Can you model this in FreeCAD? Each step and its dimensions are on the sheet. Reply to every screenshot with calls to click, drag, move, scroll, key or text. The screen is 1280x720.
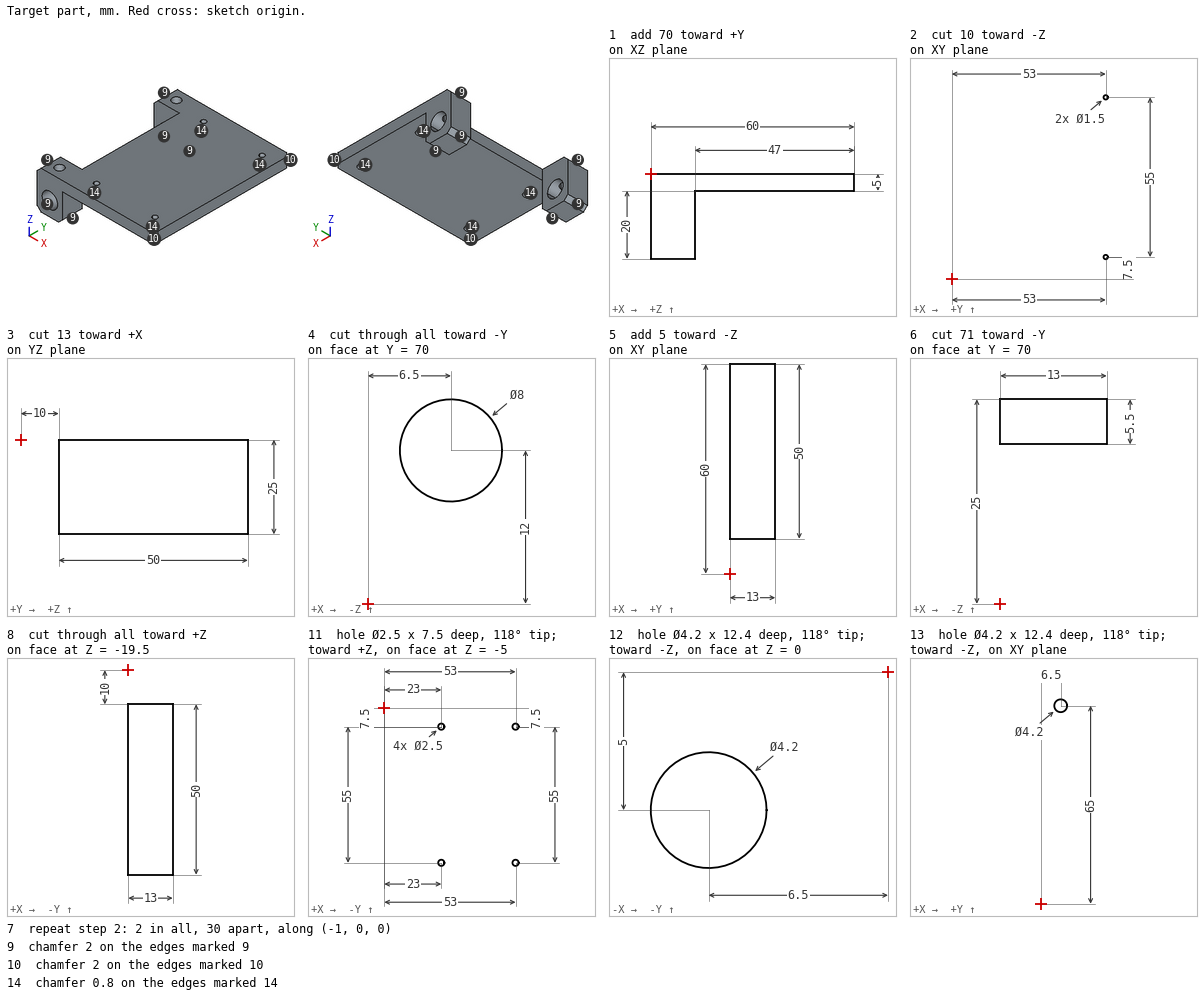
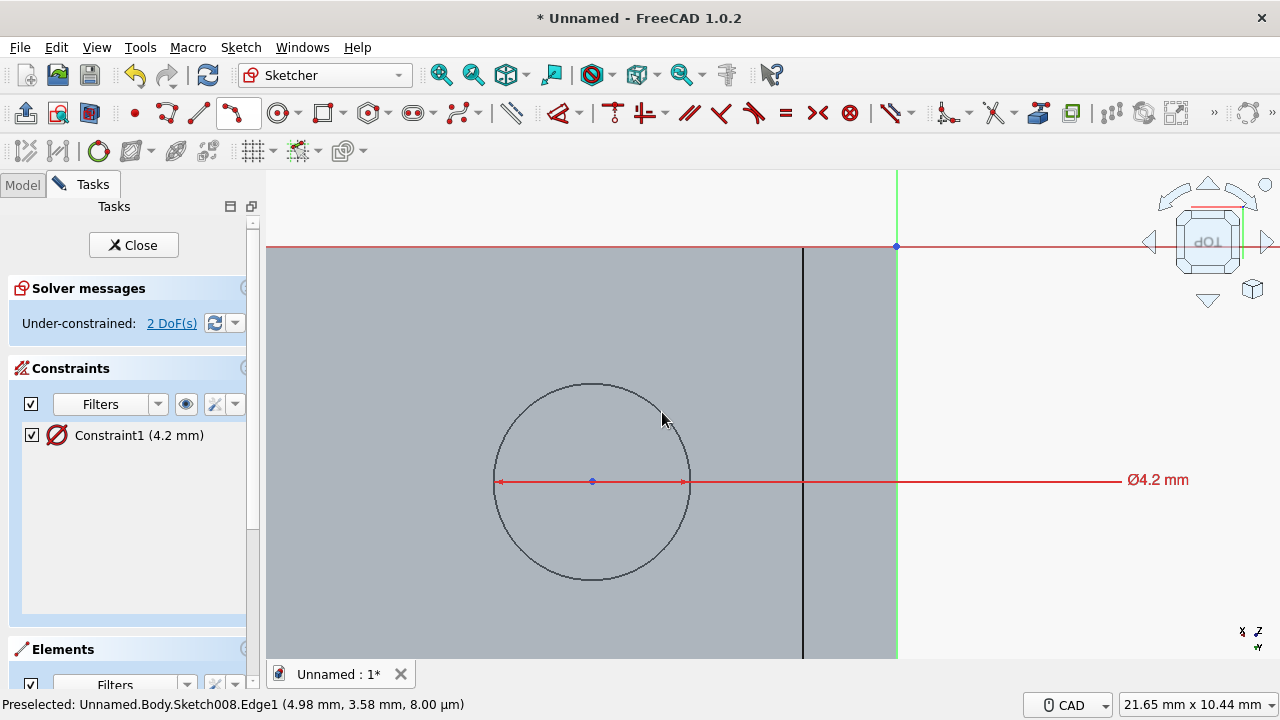
key(d)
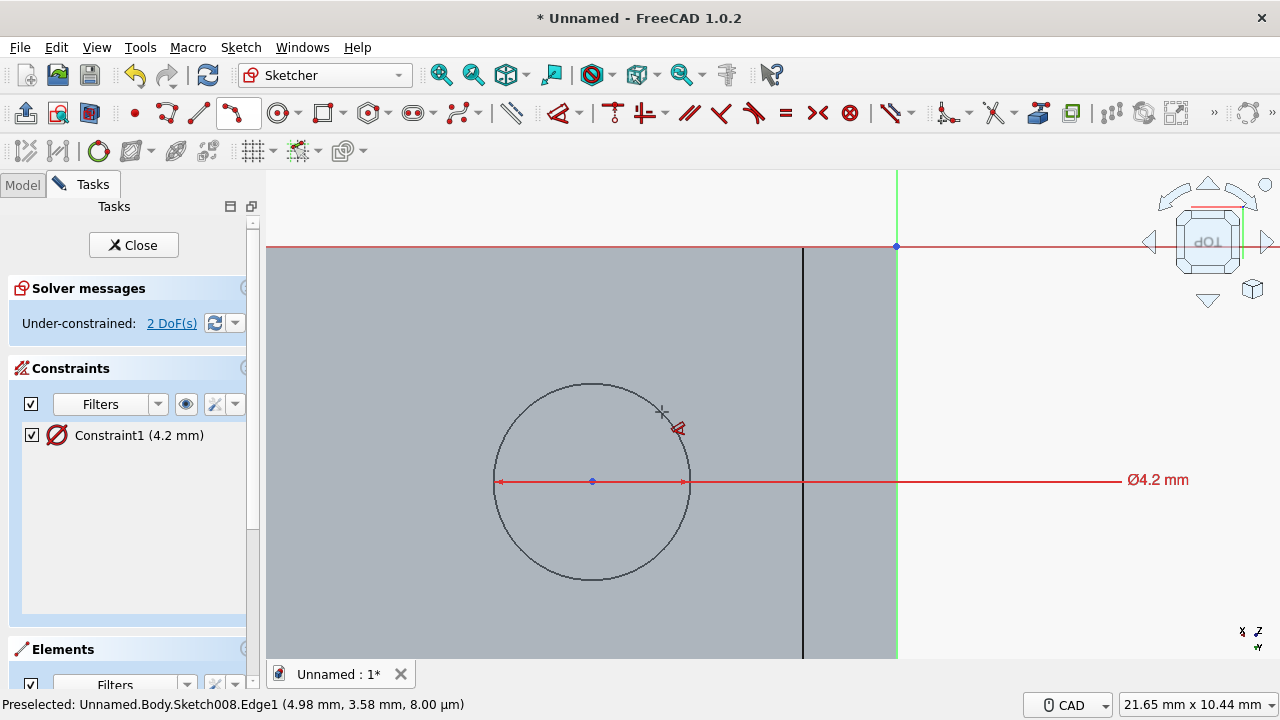
click(592, 482)
click(931, 364)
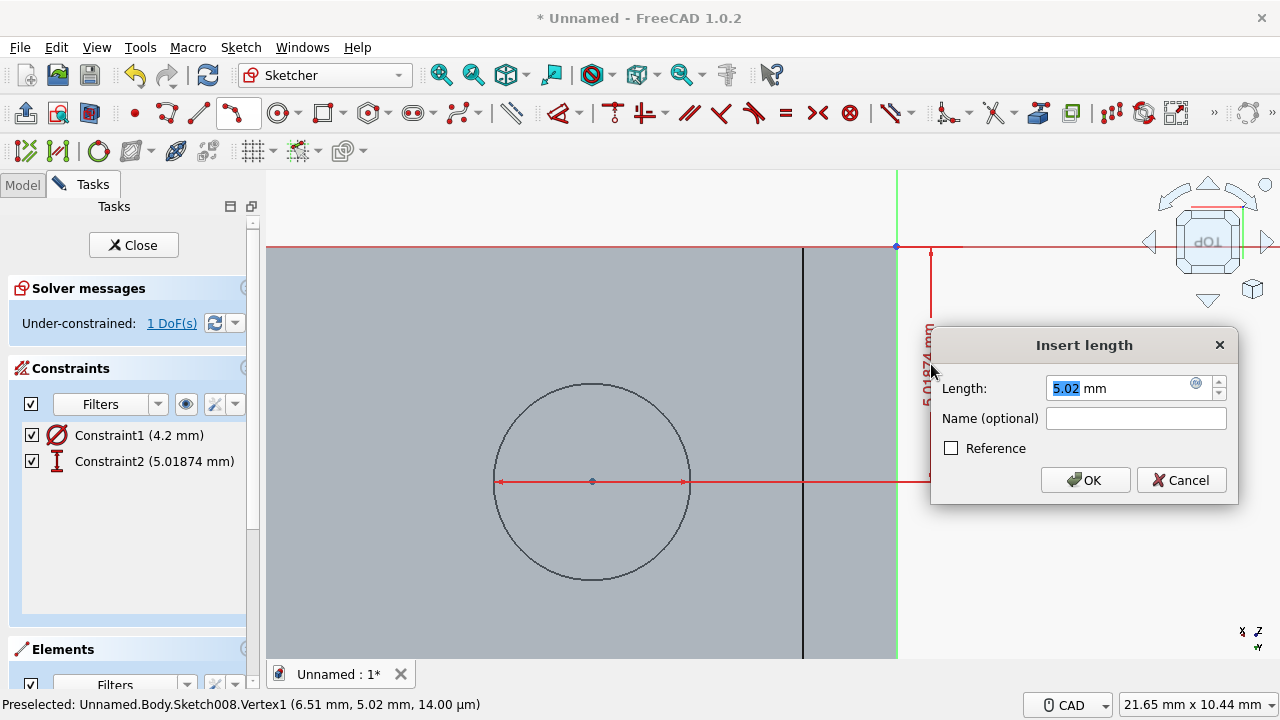
text(5)
key(Return)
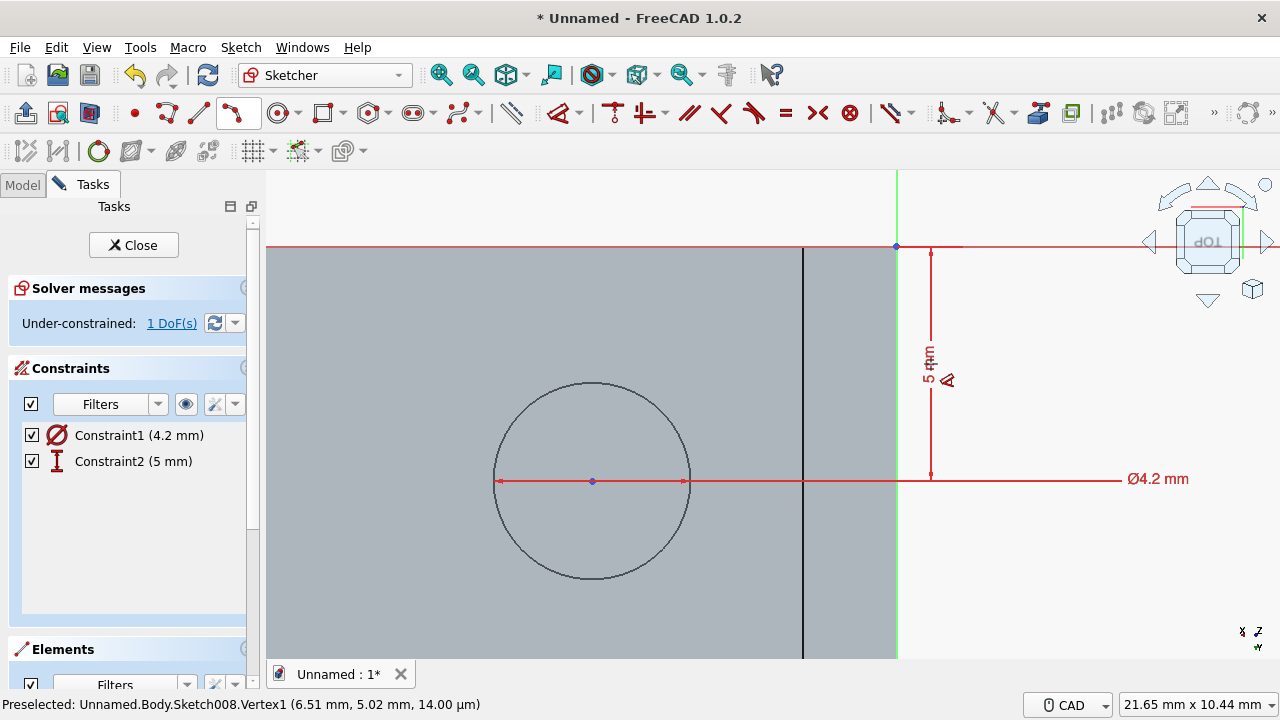
click(592, 481)
click(744, 213)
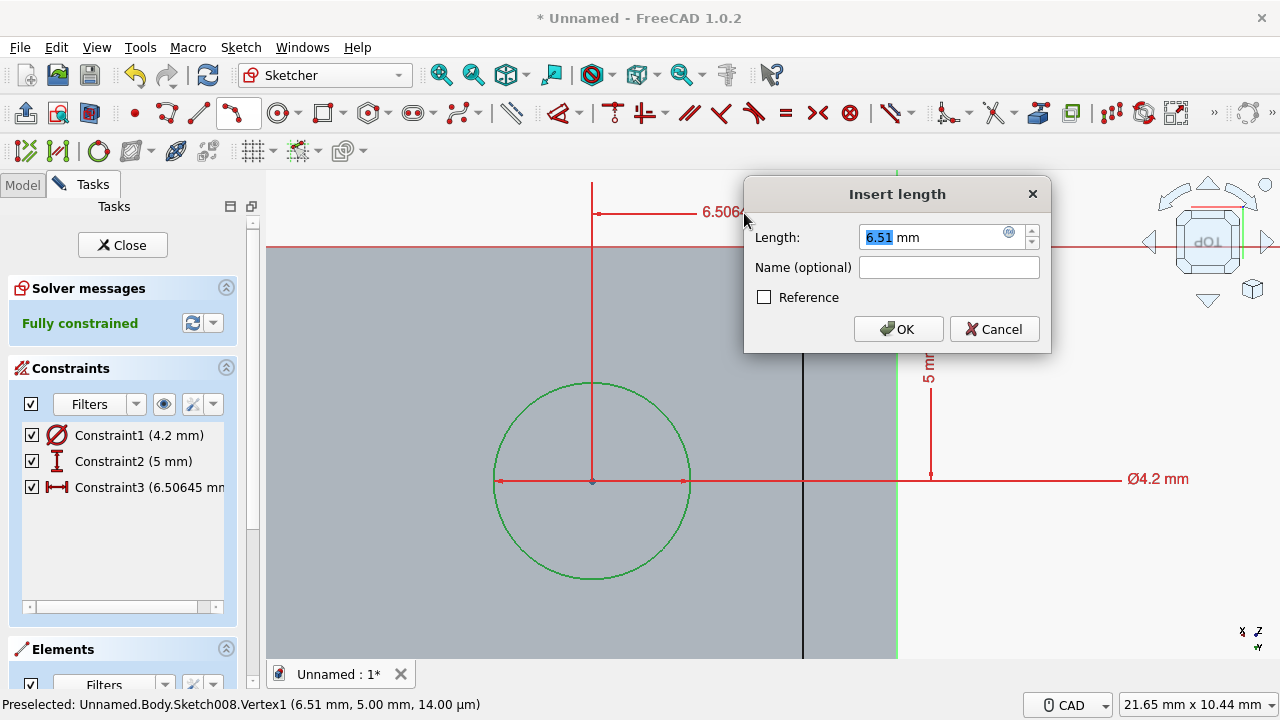
text(6.5)
key(Return)
key(Escape)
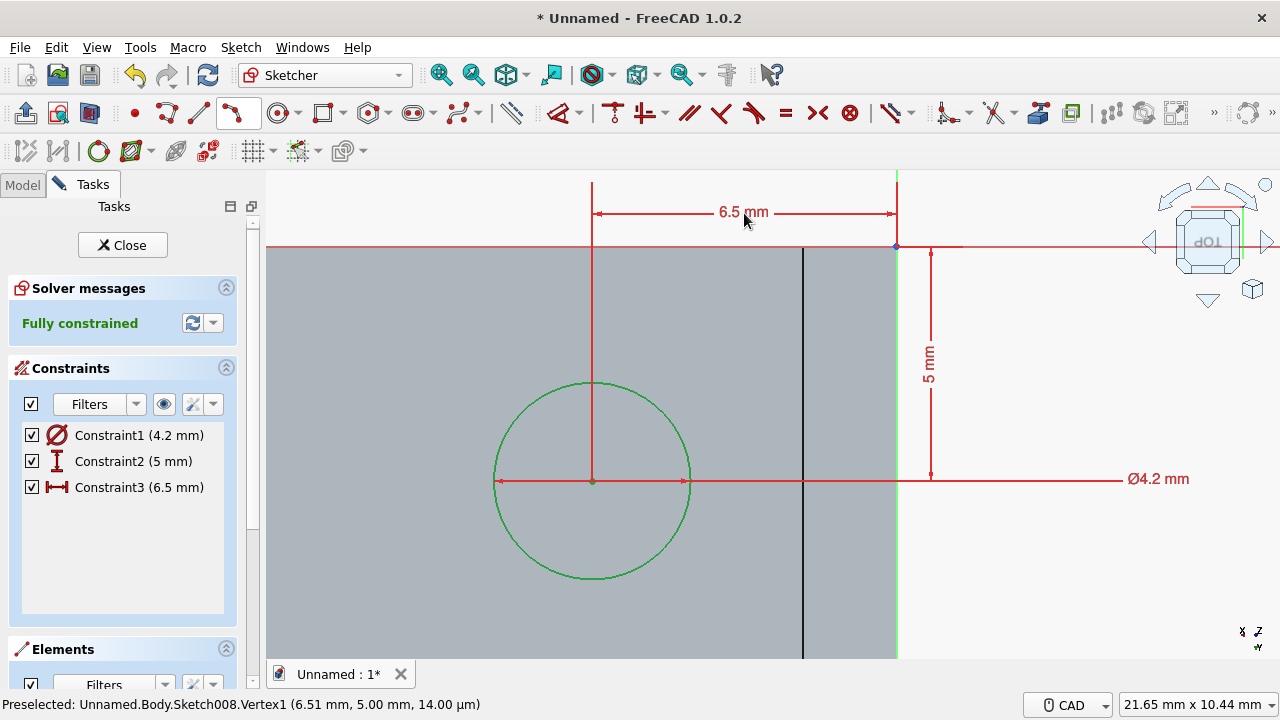
click(123, 245)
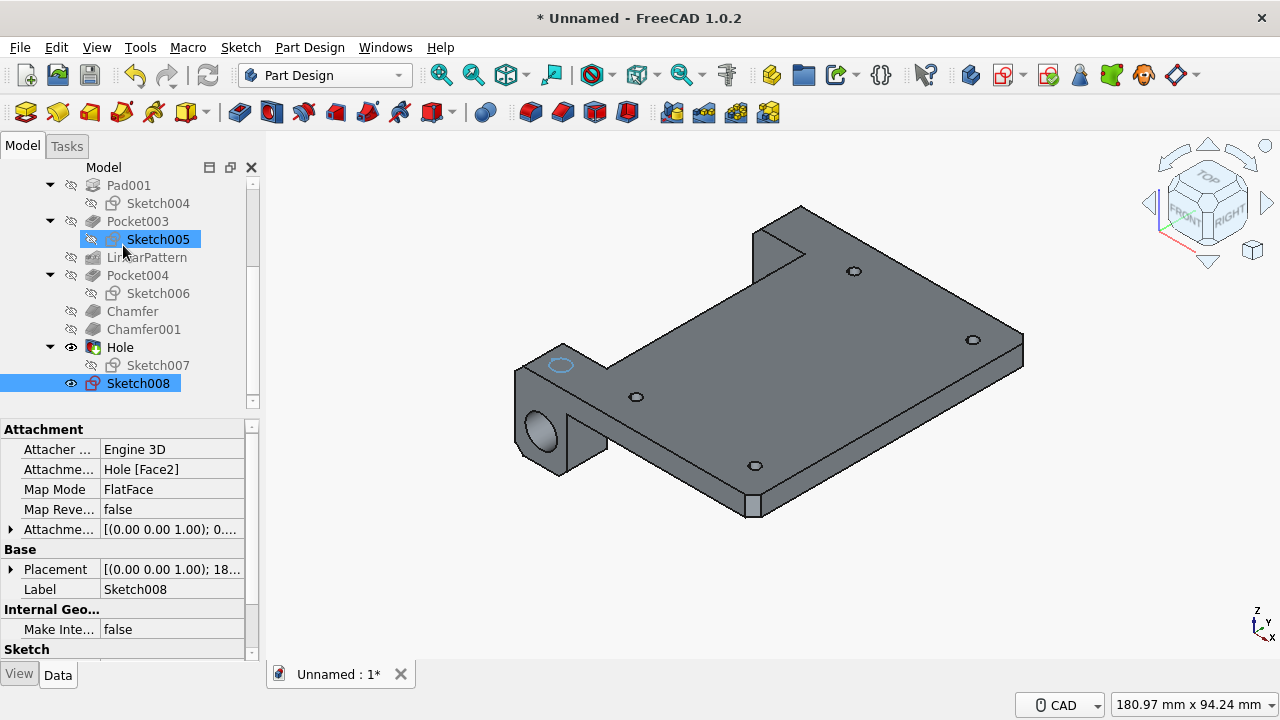
click(272, 112)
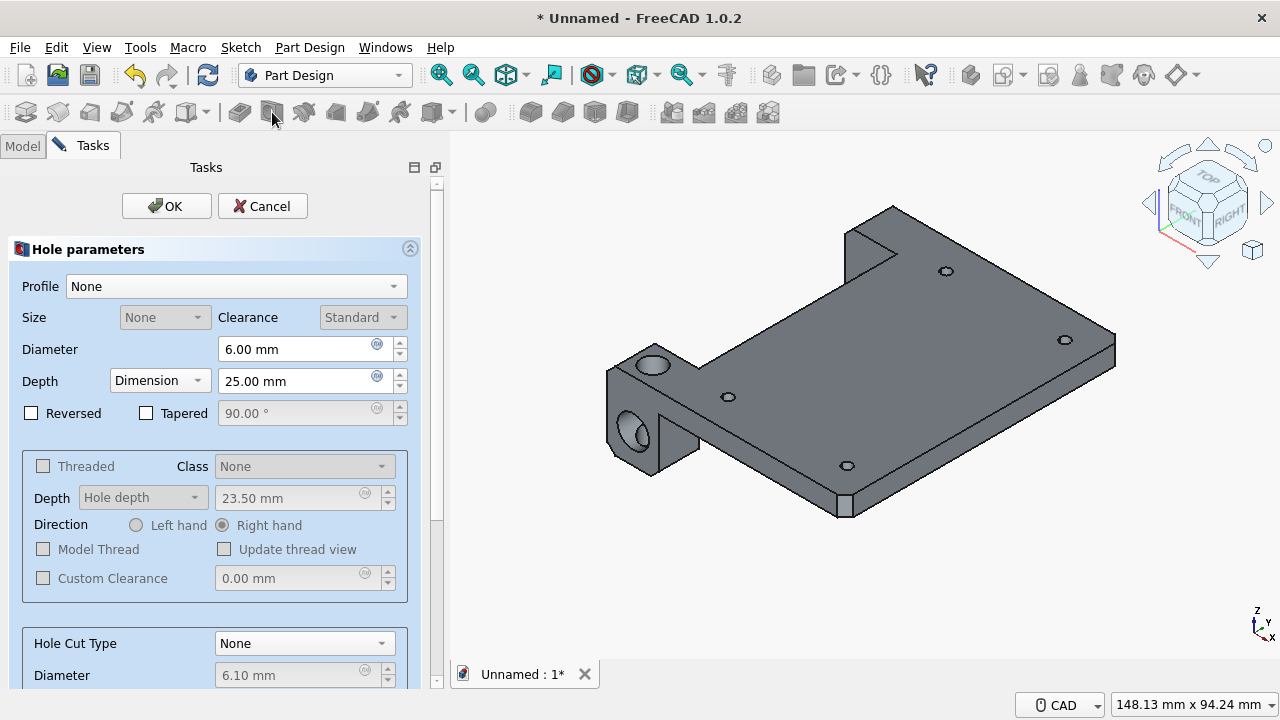
triple_click(305, 349)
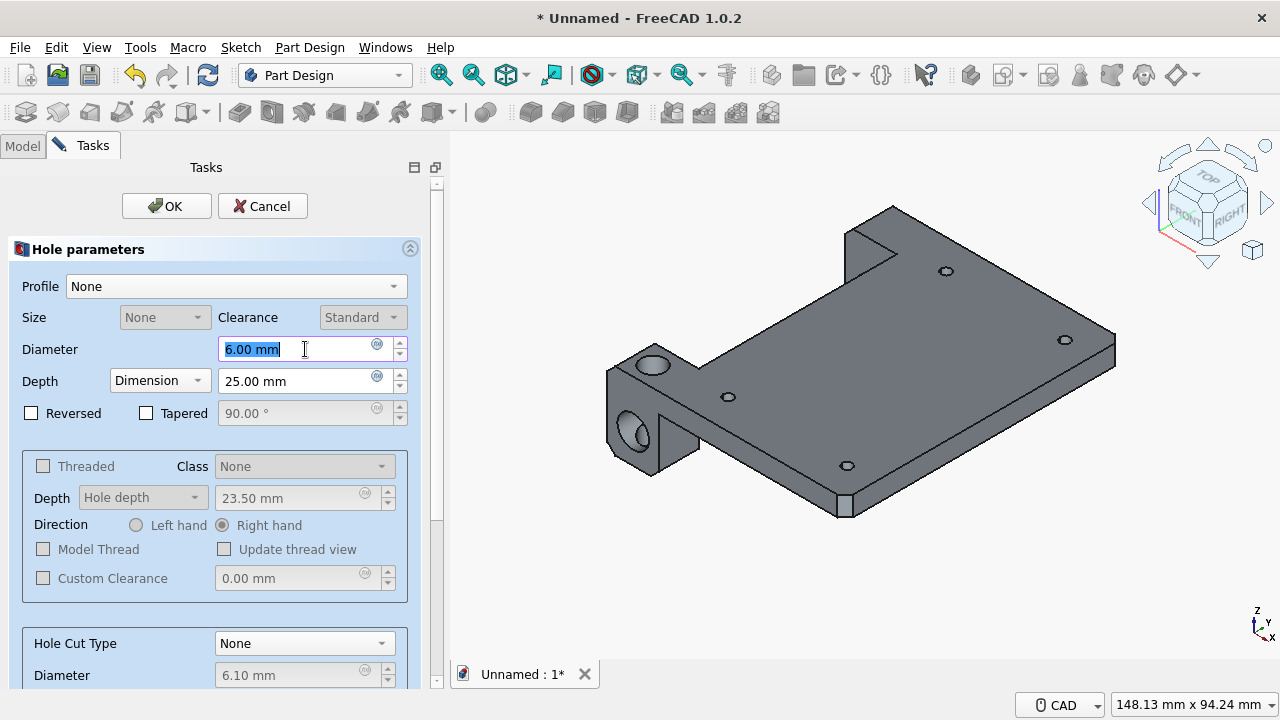
text(4.2)
key(Tab)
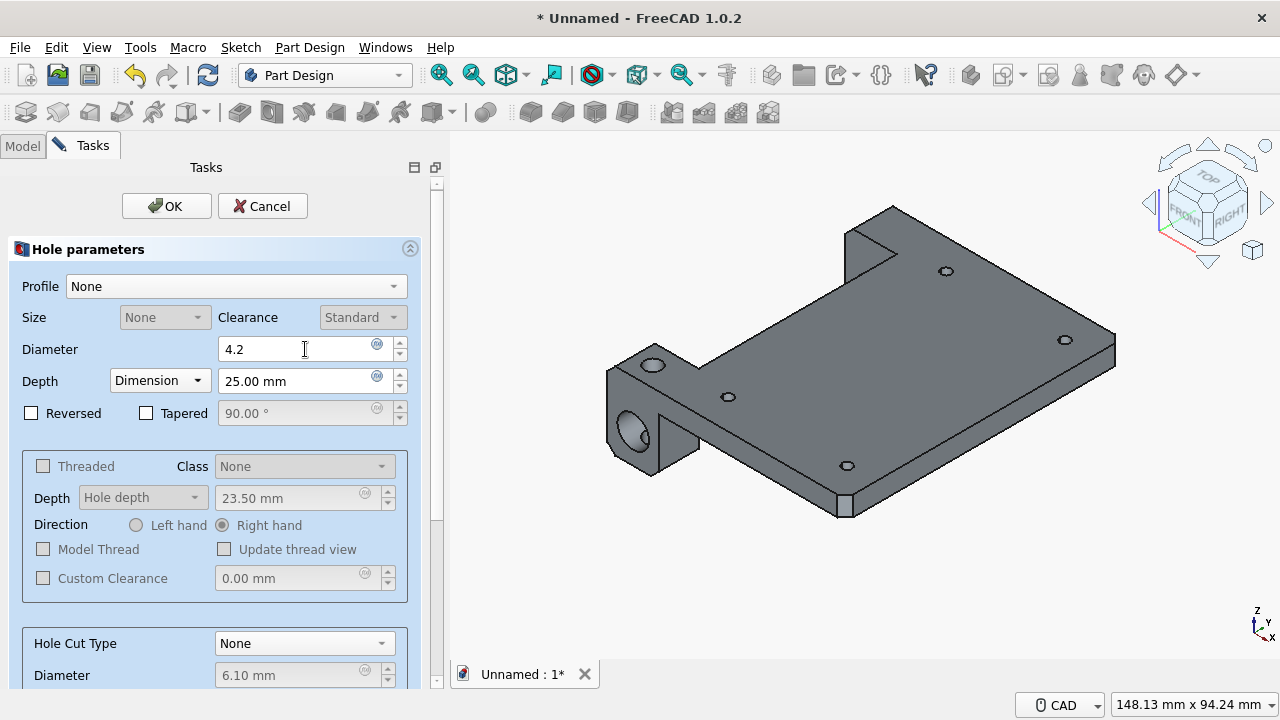
triple_click(305, 381)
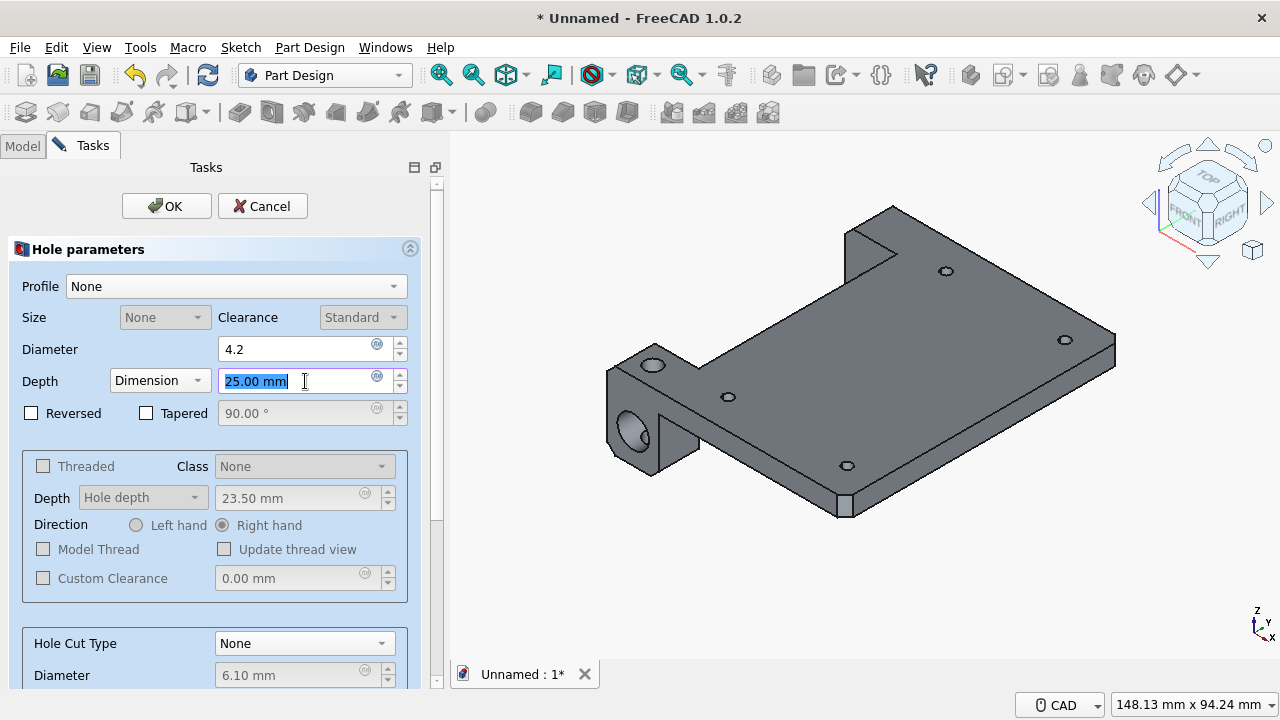
text(12.4)
key(Tab)